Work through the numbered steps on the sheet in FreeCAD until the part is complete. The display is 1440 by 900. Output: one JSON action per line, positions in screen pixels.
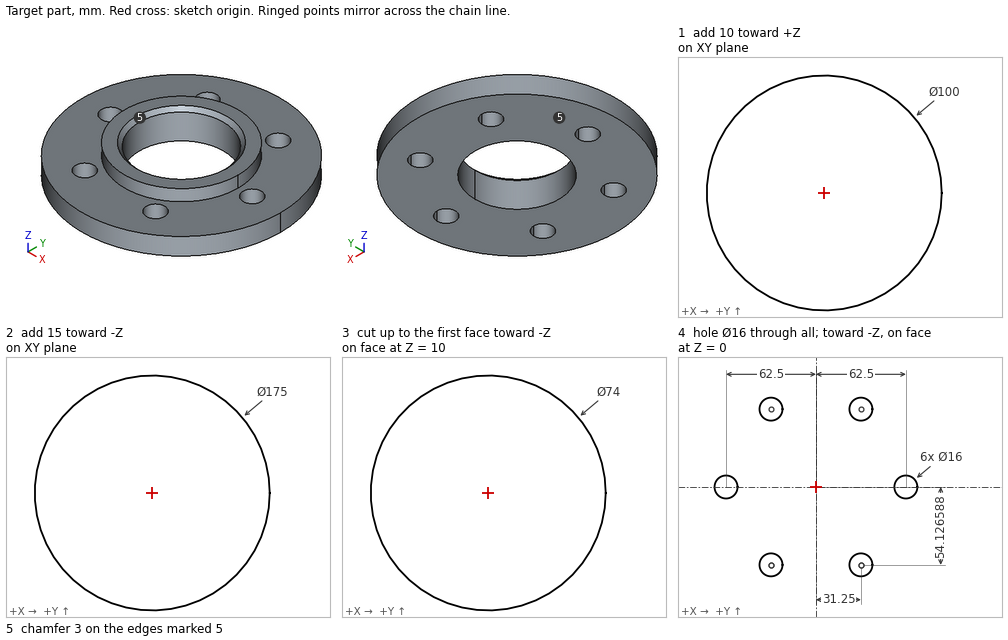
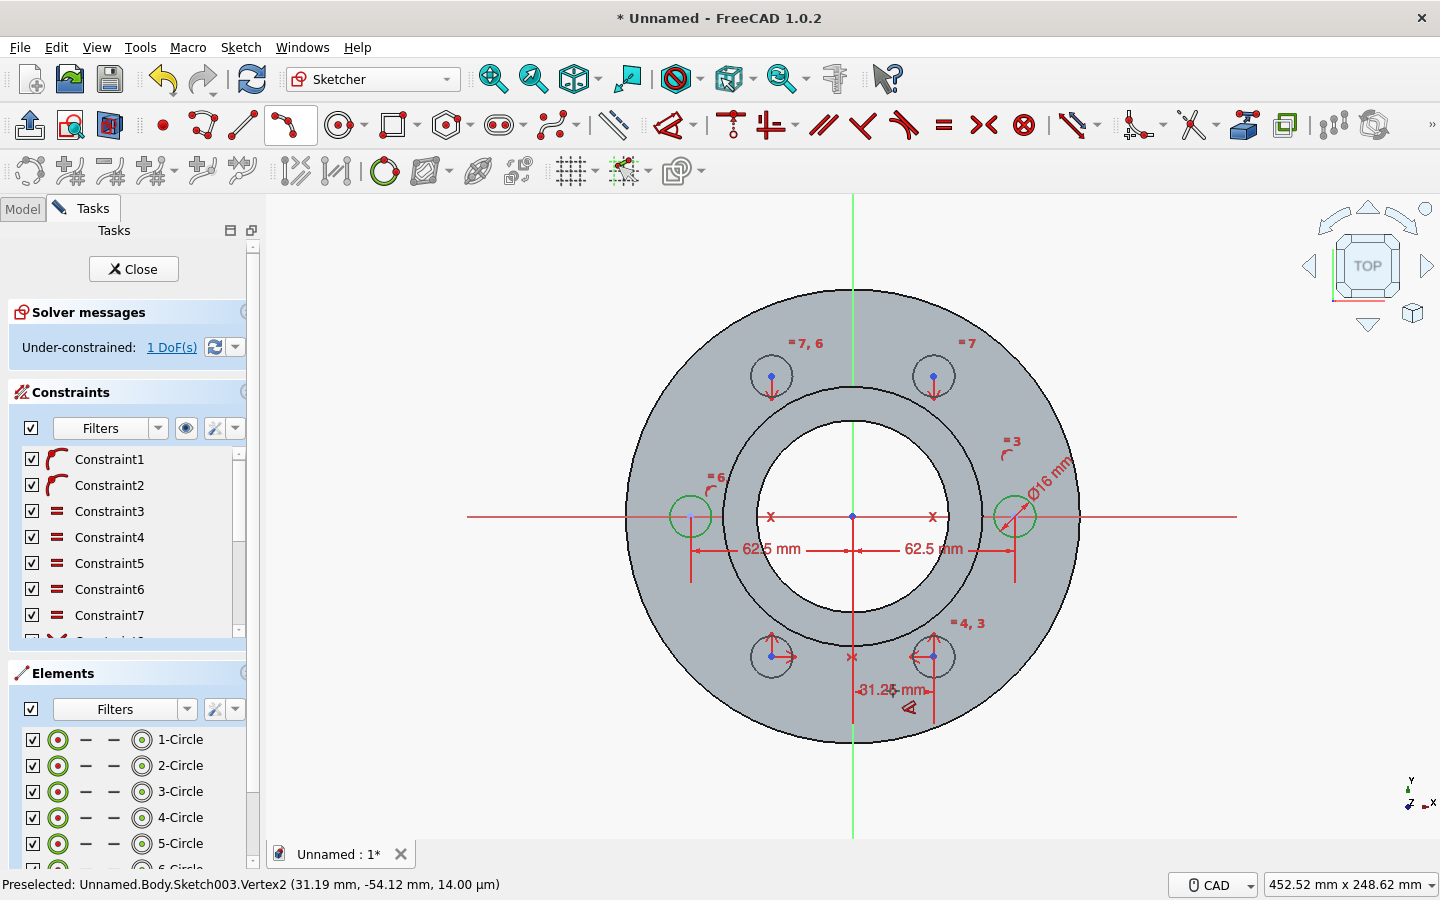
{"action": "left_click", "coordinate": [934, 657]}
{"action": "left_click", "coordinate": [968, 587]}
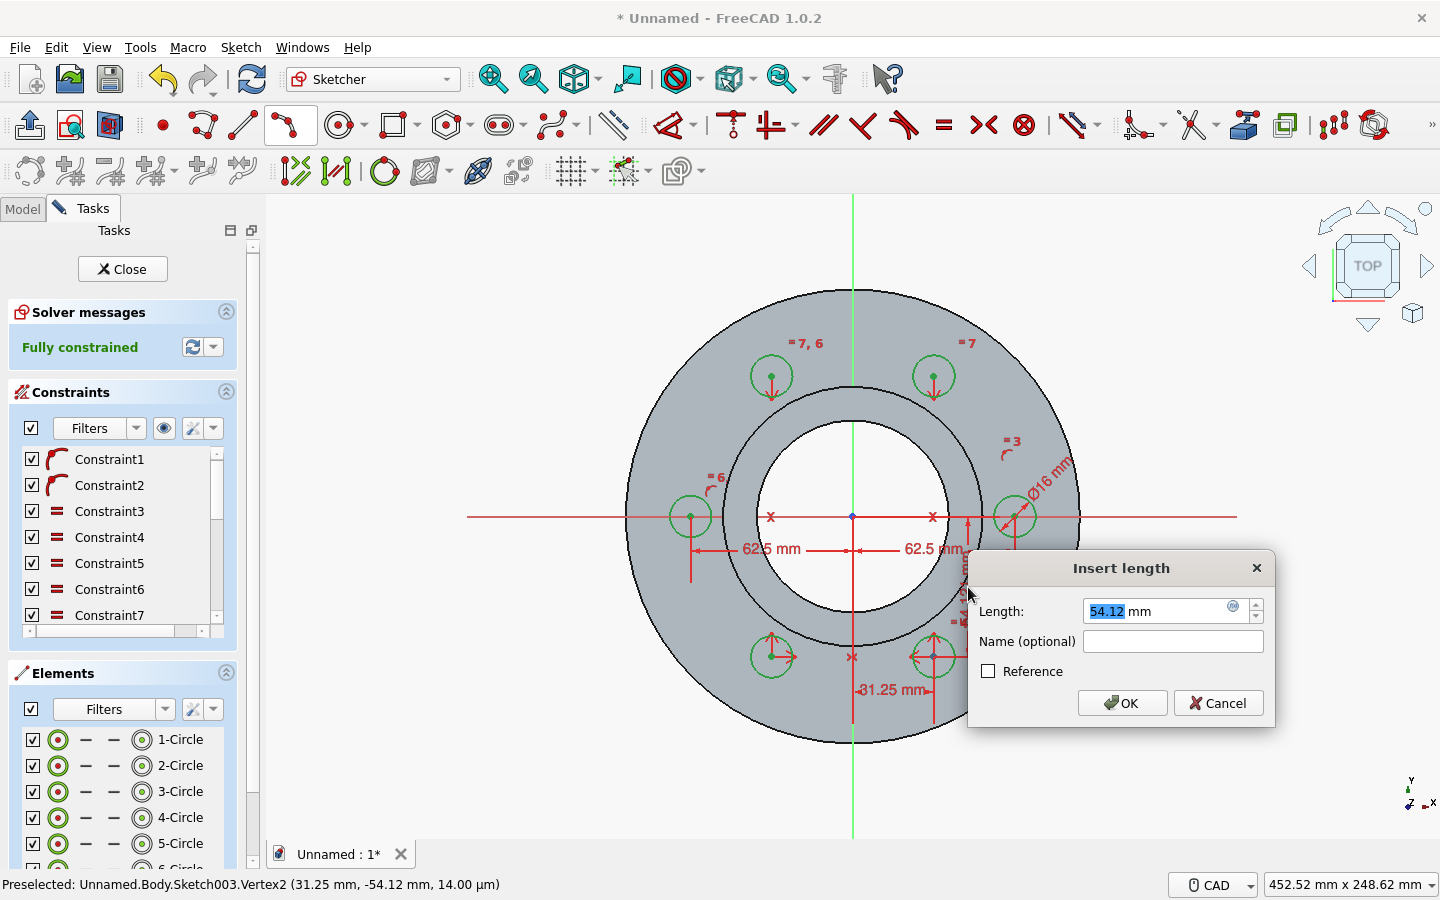
{"action": "type", "text": "54.126588"}
{"action": "key", "text": "Return"}
{"action": "key", "text": "Escape"}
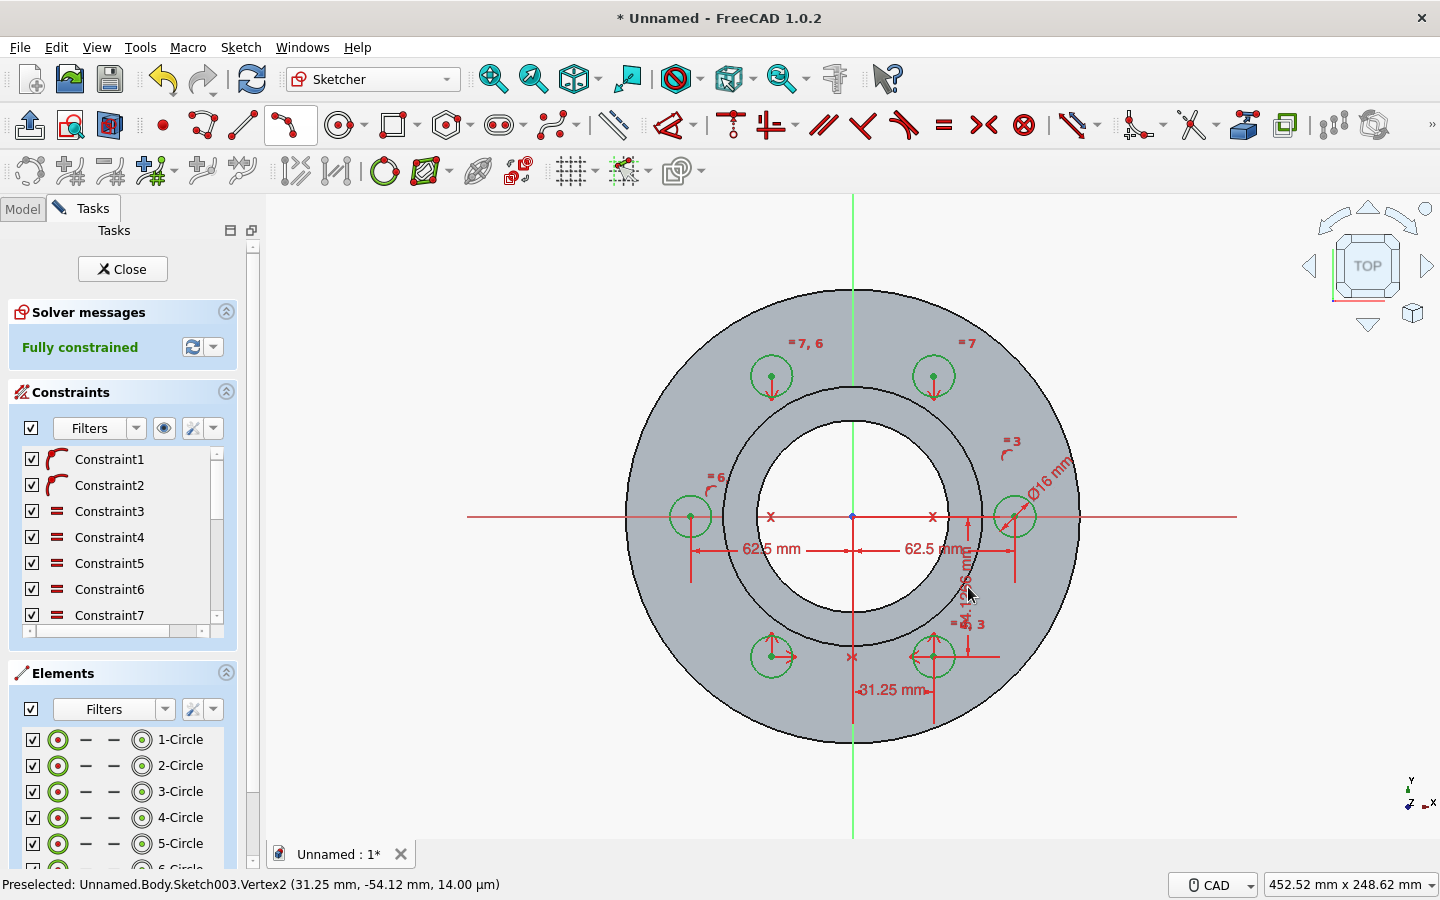
{"action": "left_click", "coordinate": [123, 269]}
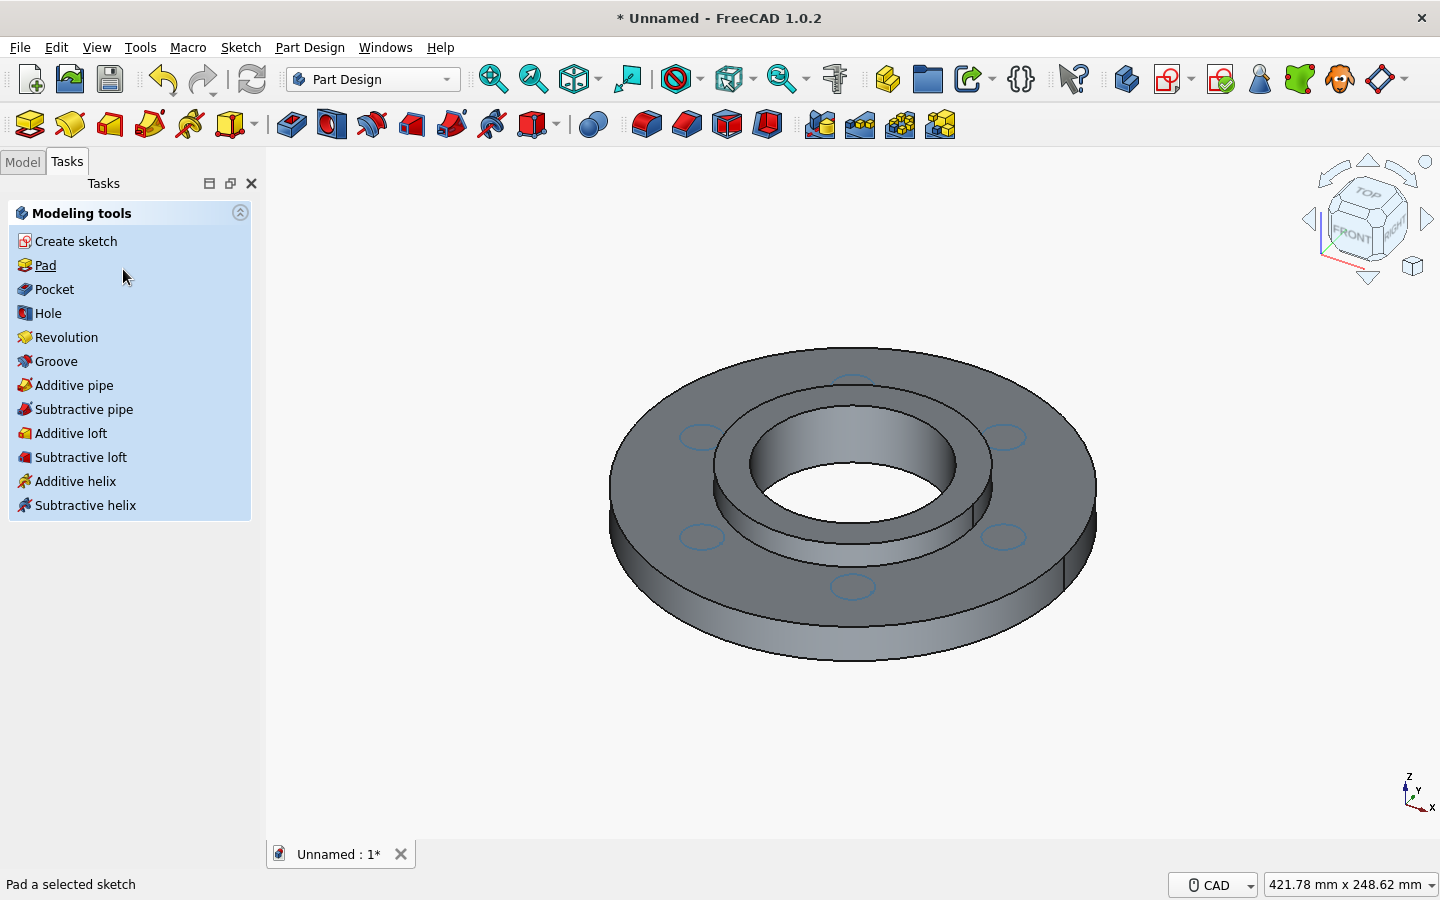
{"action": "left_click", "coordinate": [332, 124]}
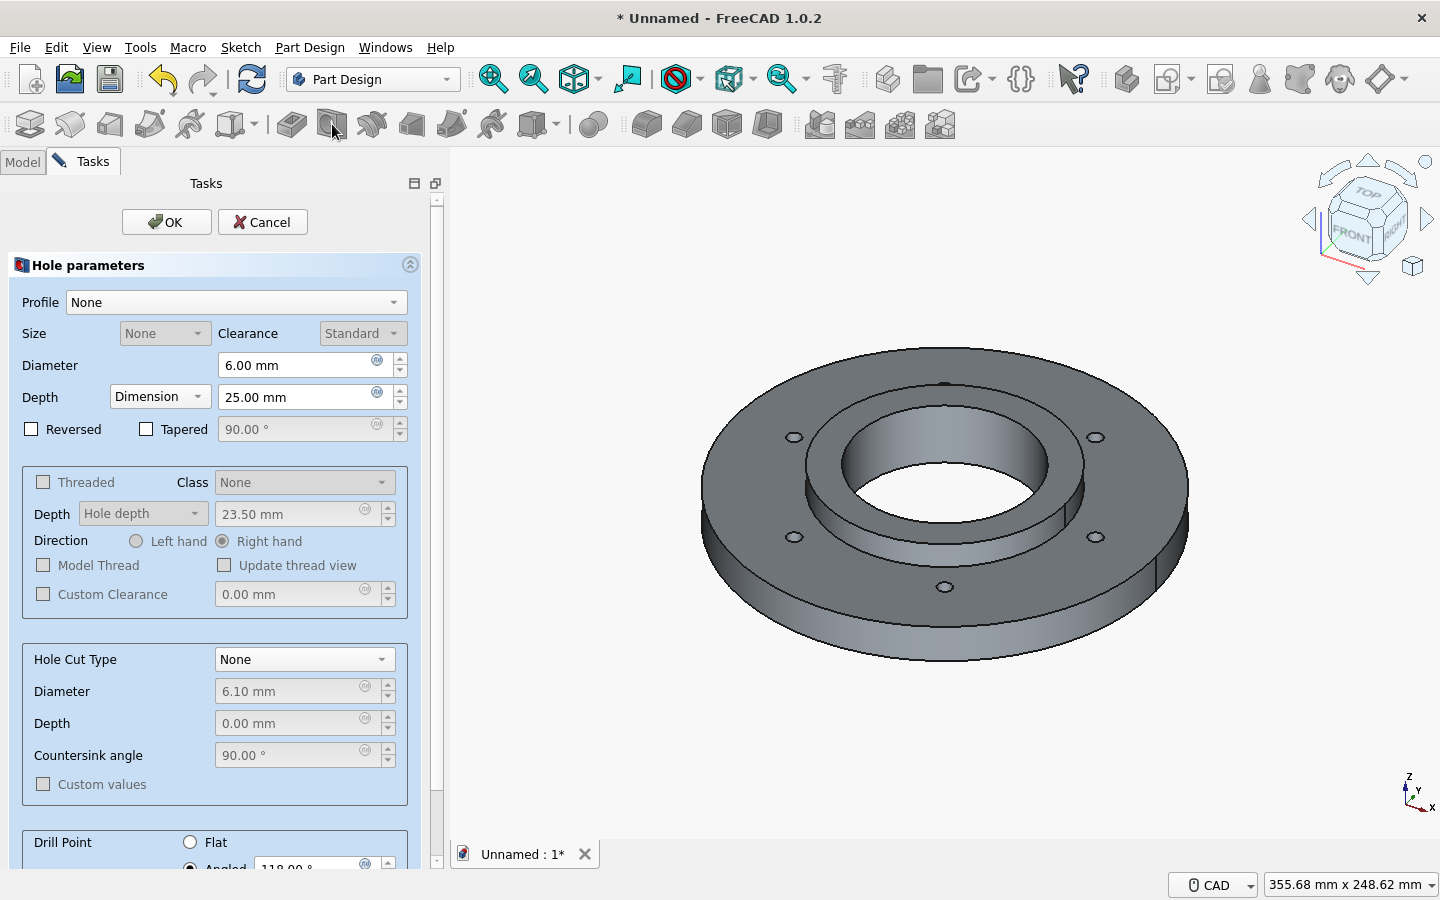
{"action": "triple_click", "coordinate": [305, 365]}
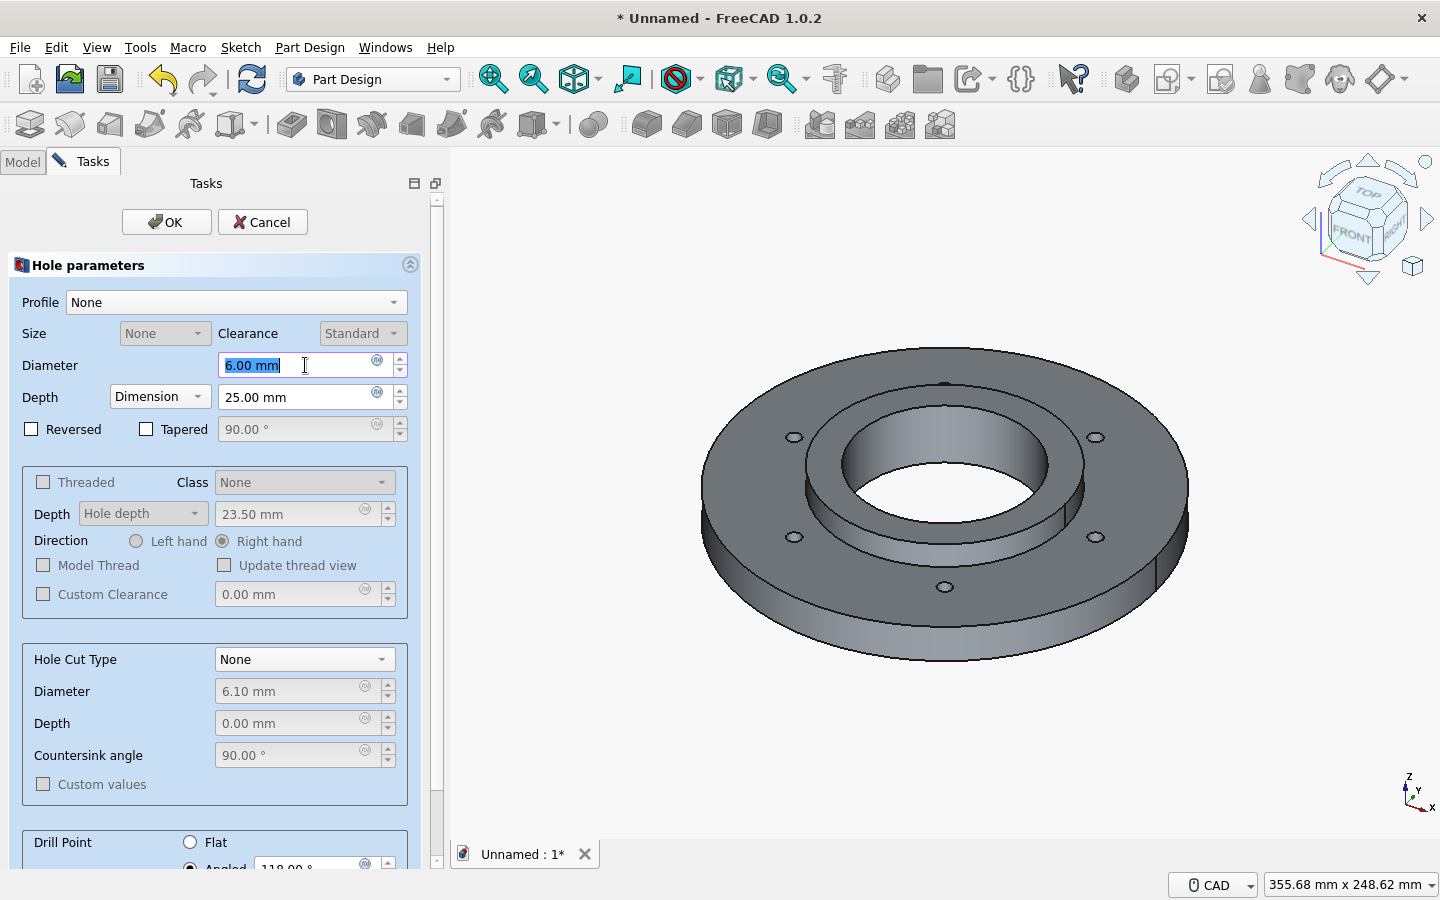
{"action": "type", "text": "16"}
{"action": "key", "text": "Tab"}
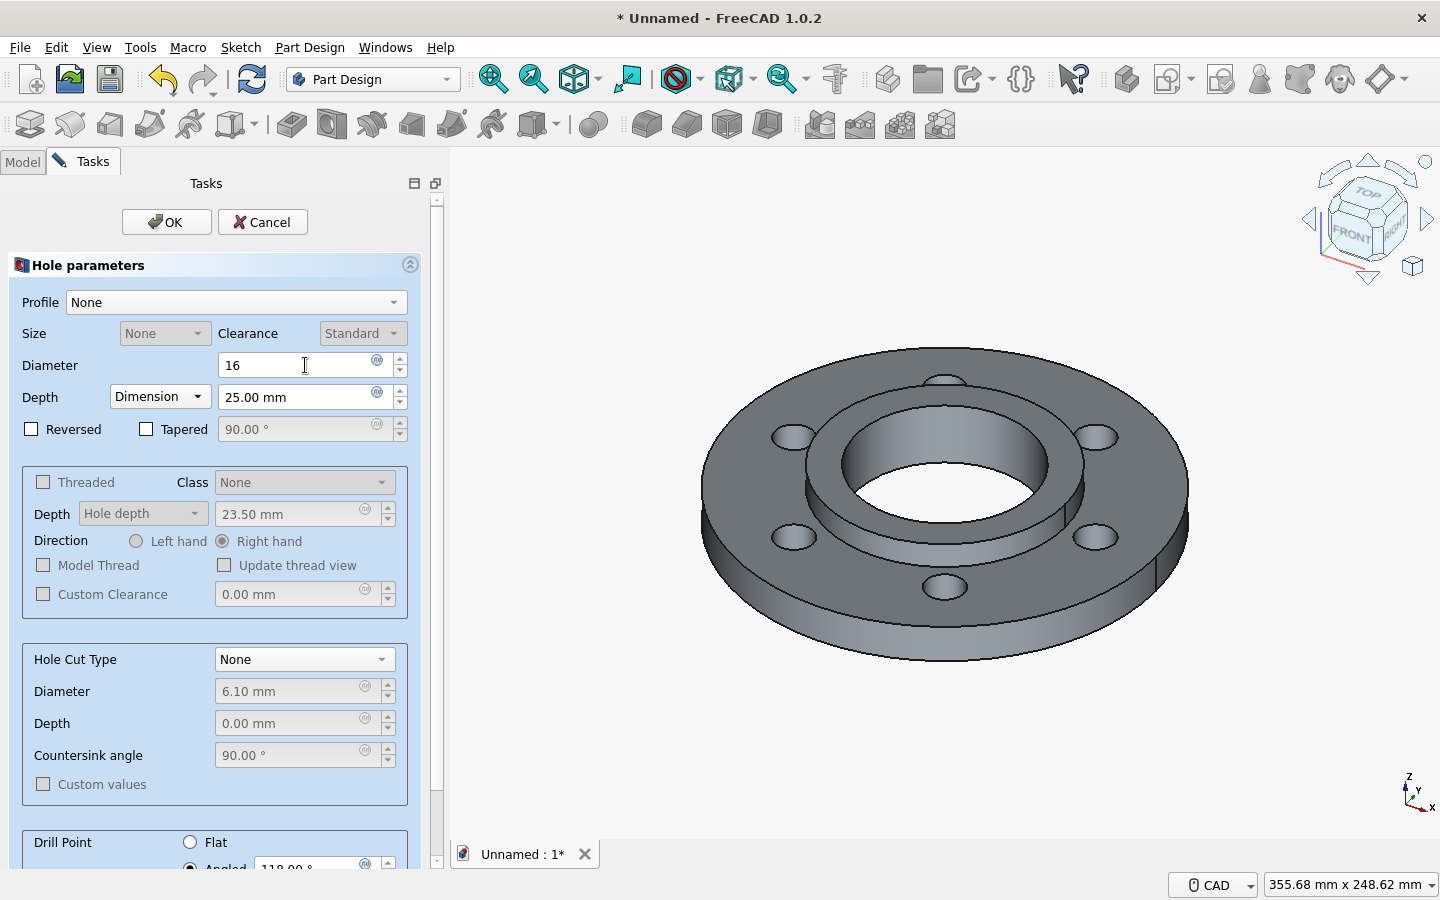
{"action": "left_click", "coordinate": [161, 396]}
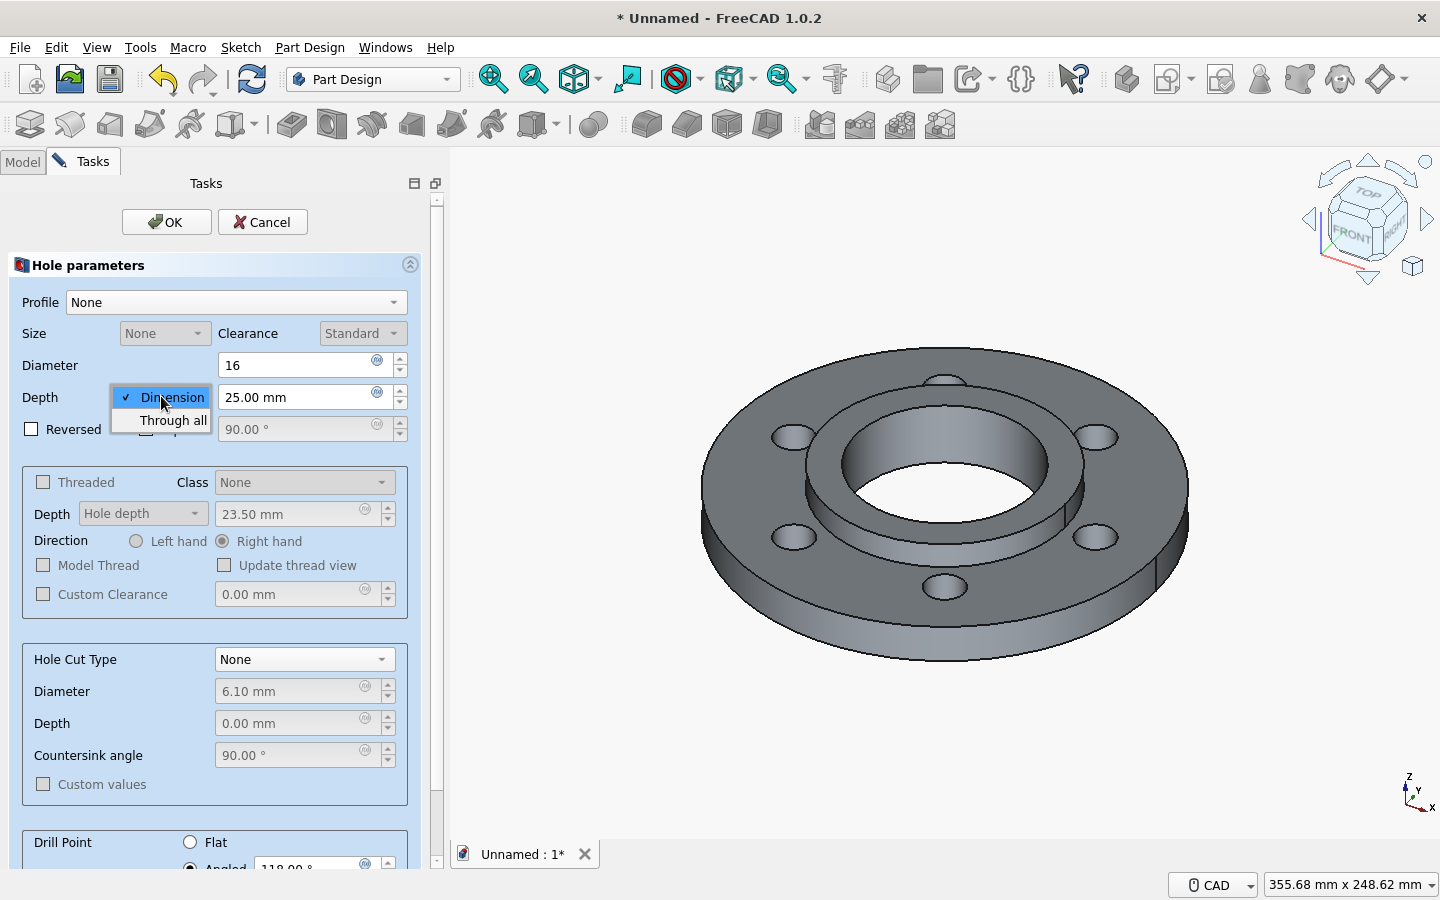
{"action": "left_click", "coordinate": [160, 420]}